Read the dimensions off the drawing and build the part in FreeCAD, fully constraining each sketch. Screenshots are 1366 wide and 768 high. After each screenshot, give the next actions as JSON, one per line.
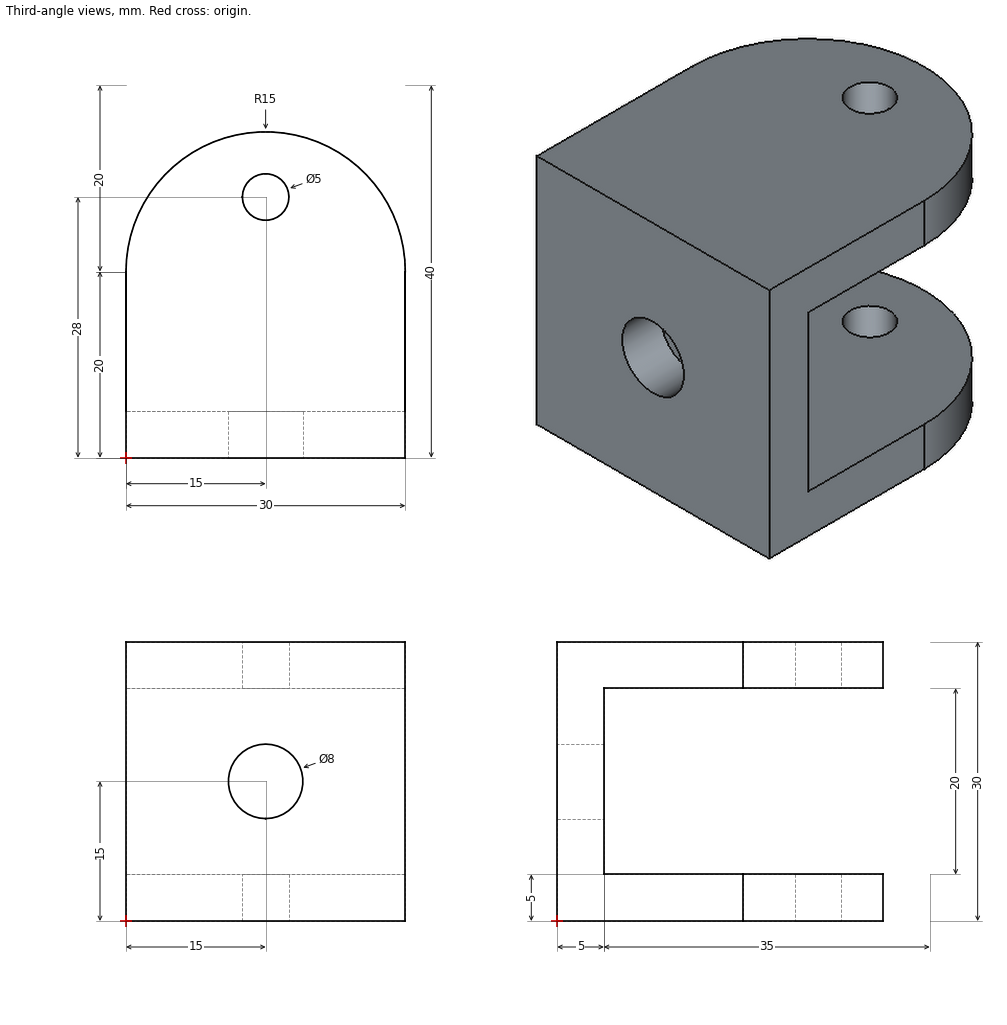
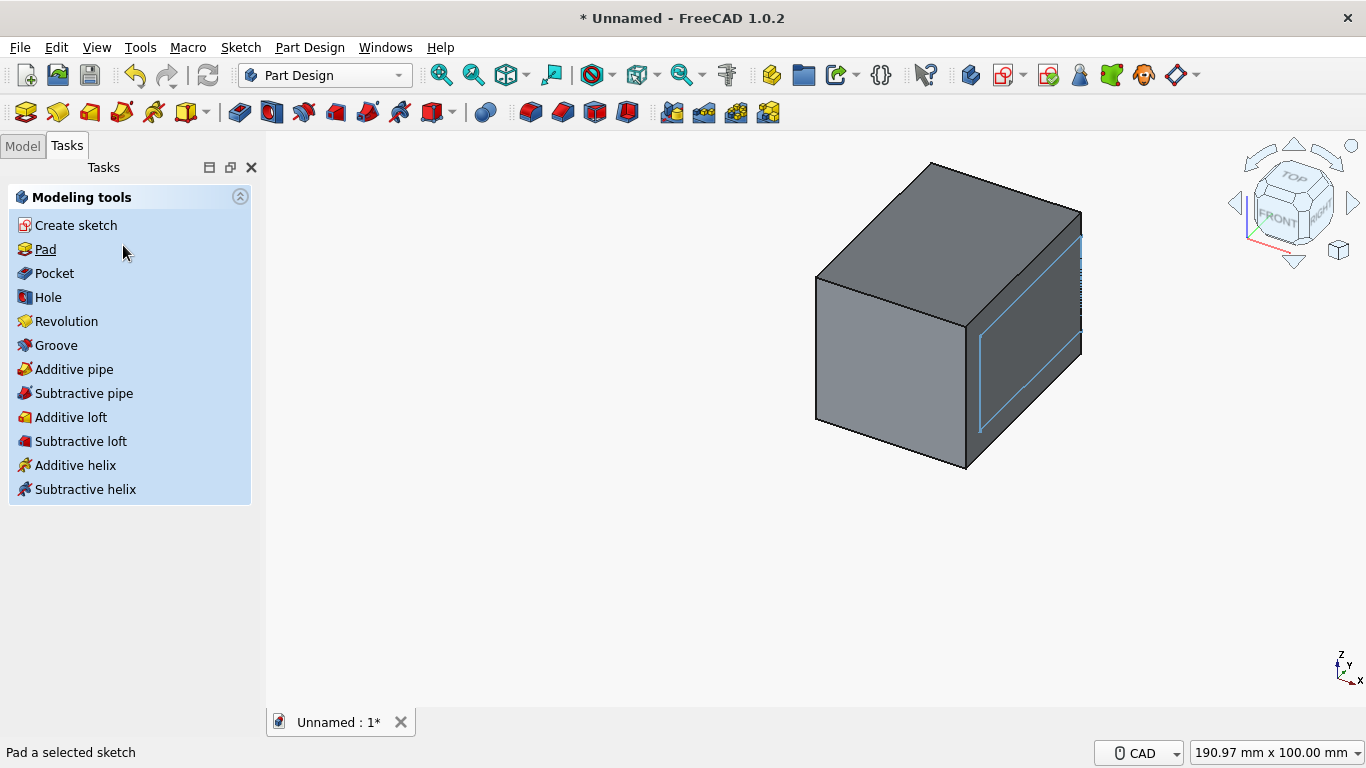
{"action": "left_click", "coordinate": [240, 112]}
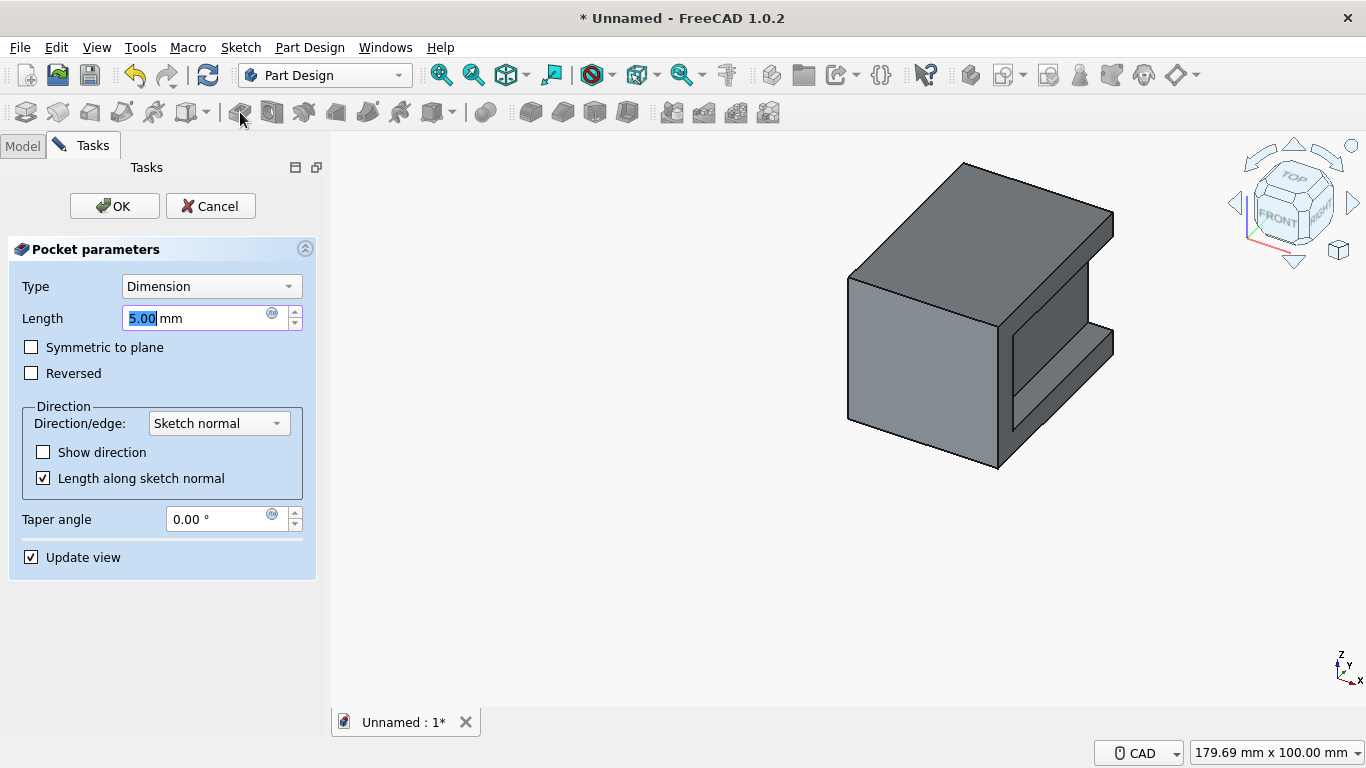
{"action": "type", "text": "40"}
{"action": "key", "text": "Tab"}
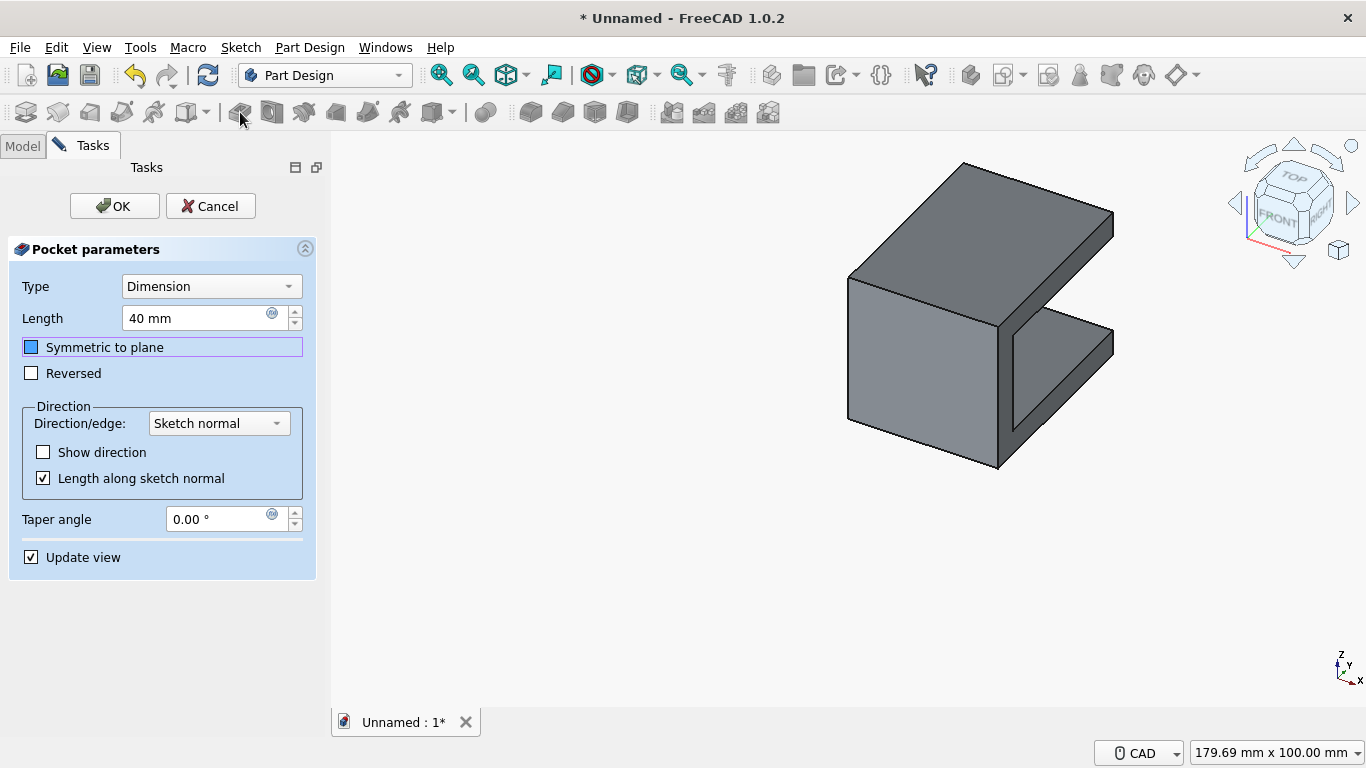
{"action": "left_click", "coordinate": [115, 206]}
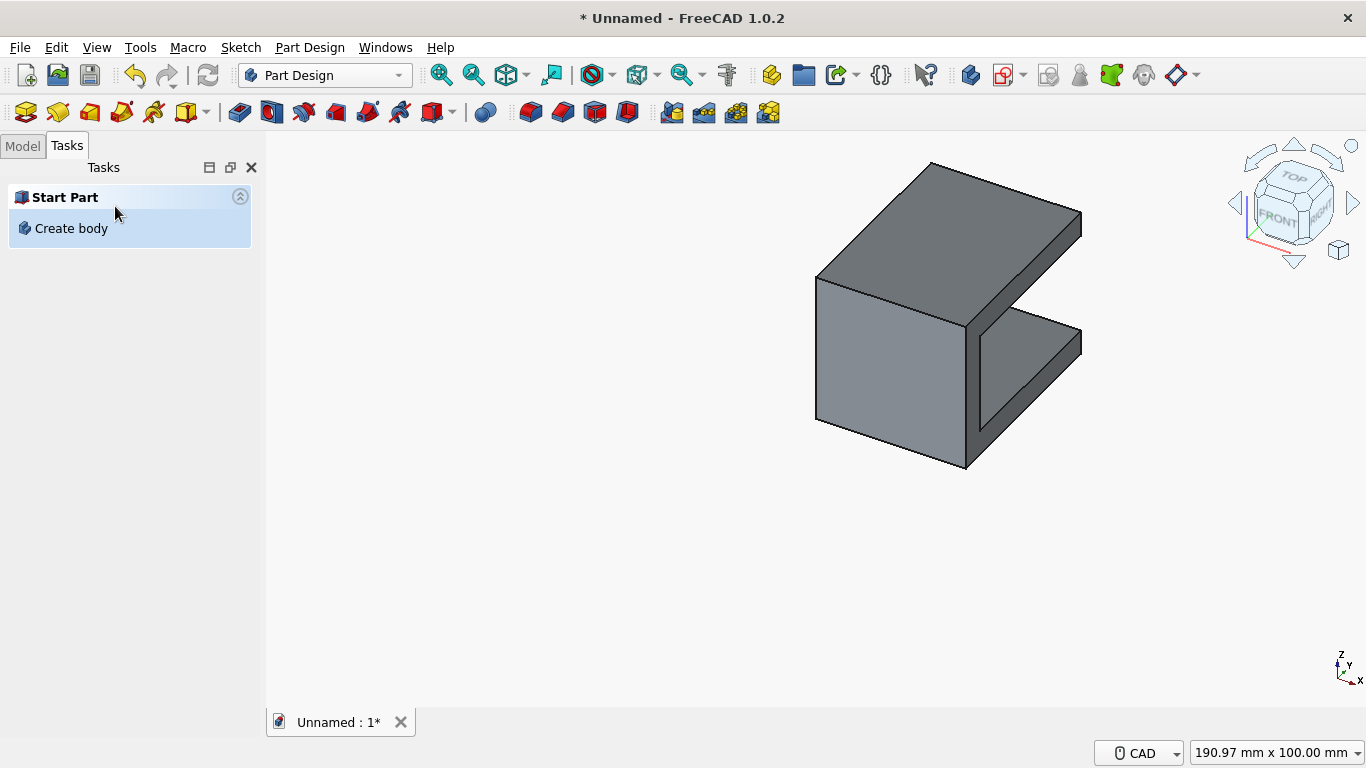
{"action": "left_click", "coordinate": [1004, 76]}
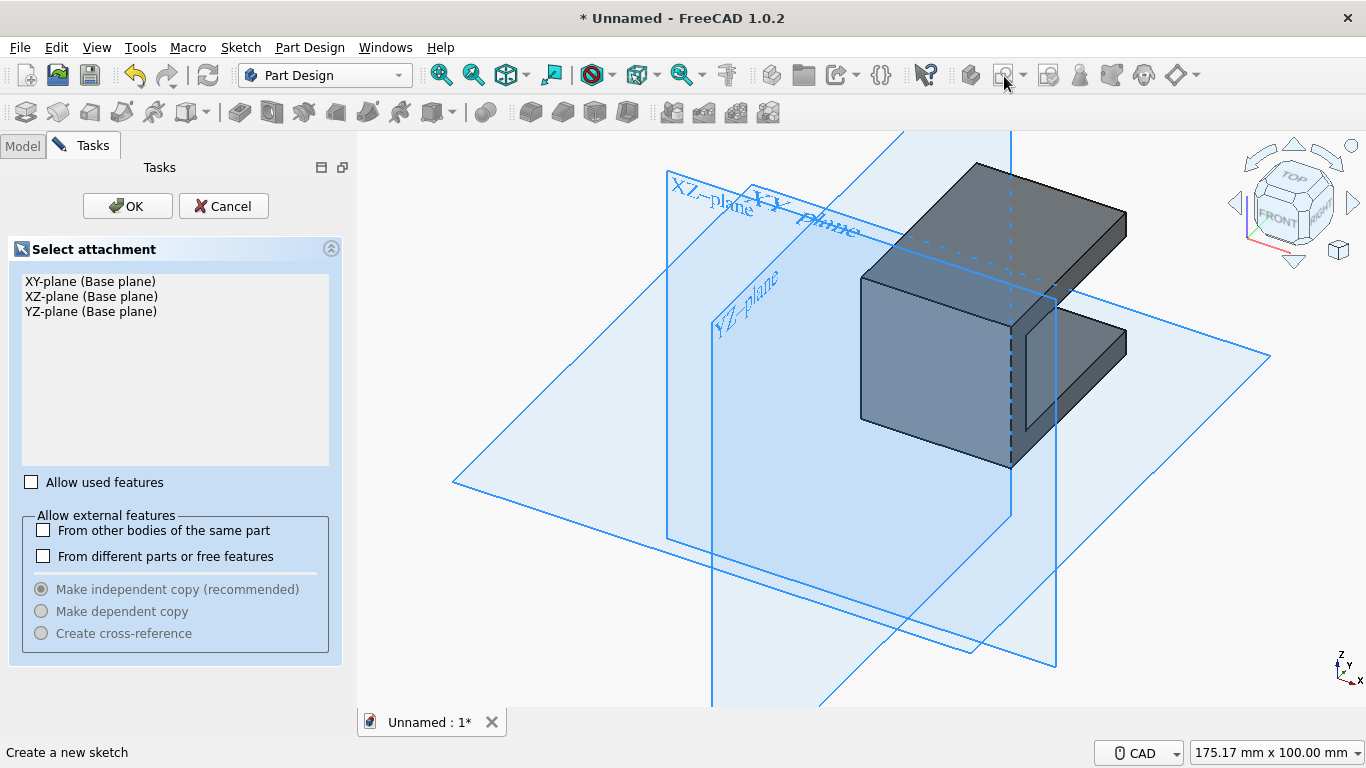
{"action": "left_click", "coordinate": [82, 282]}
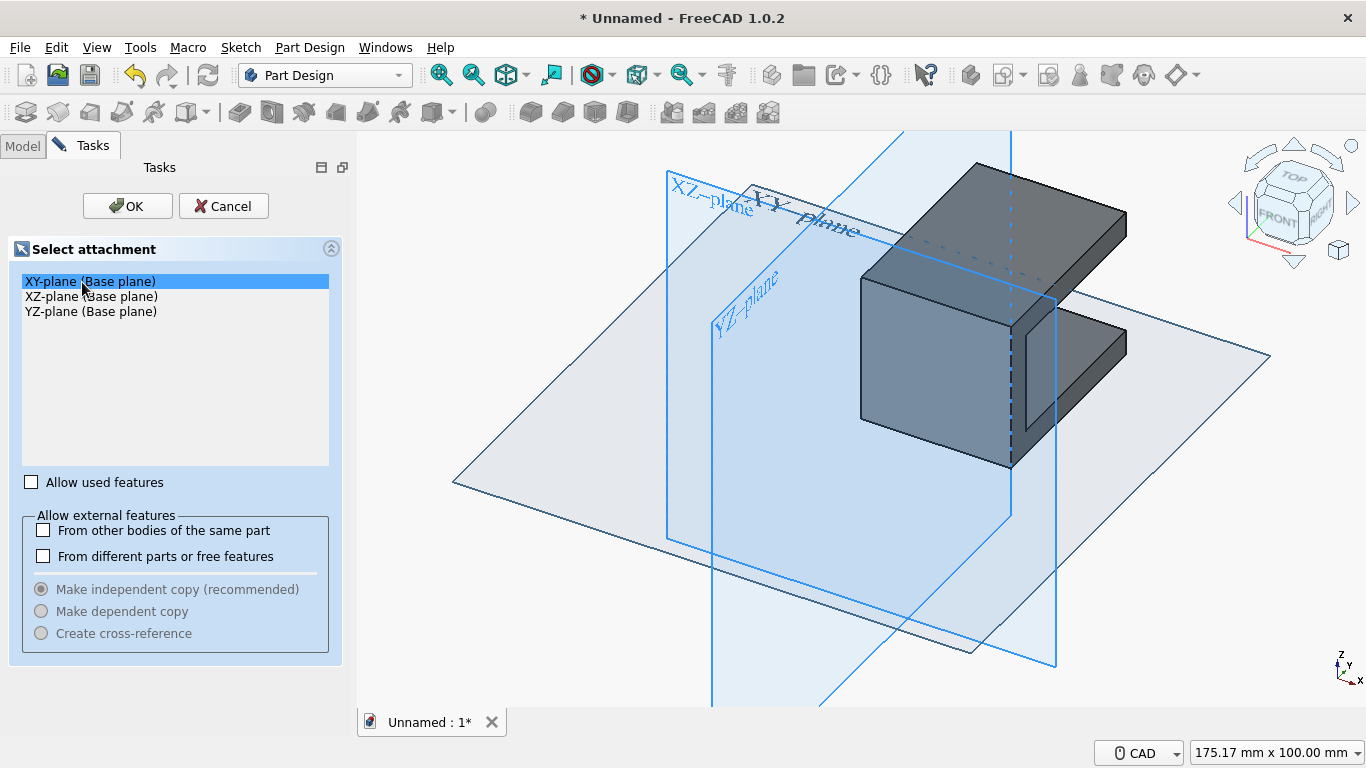
{"action": "left_click", "coordinate": [128, 206]}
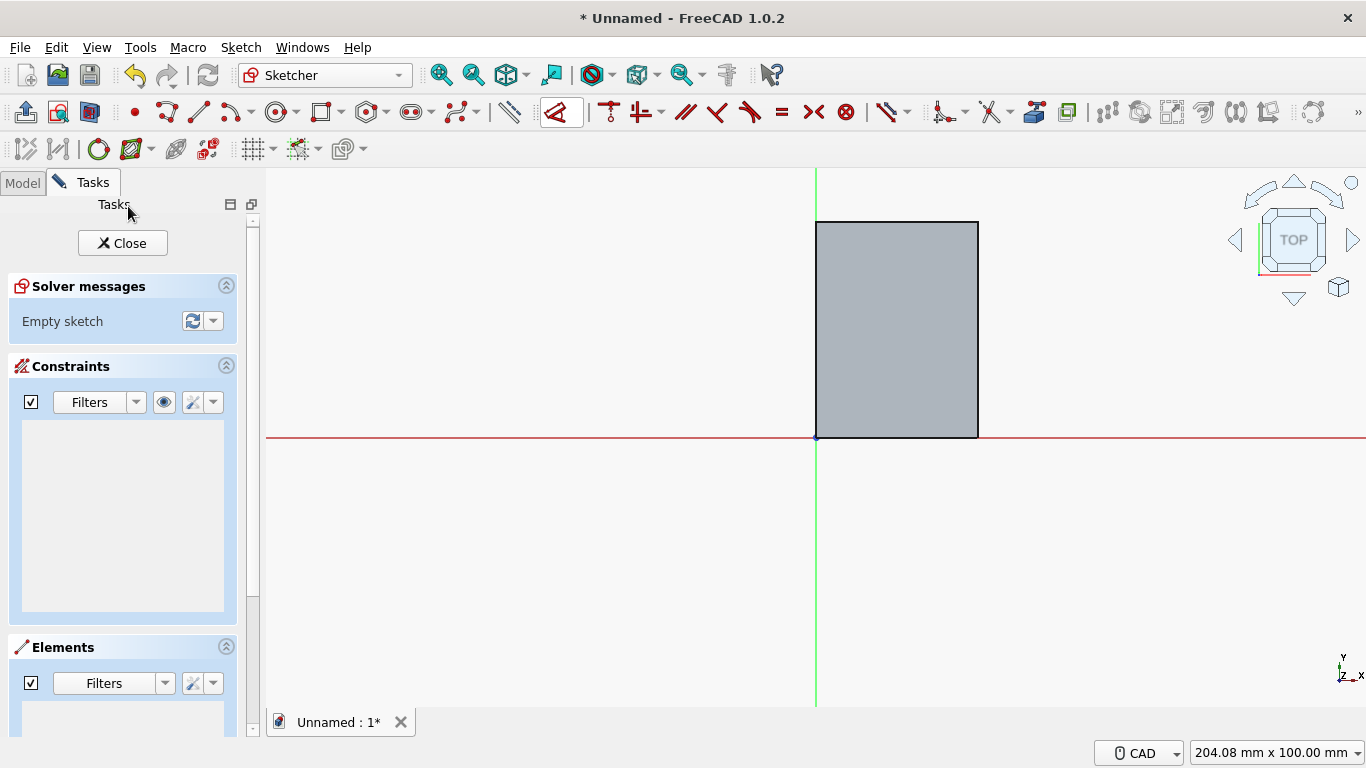
{"action": "left_click", "coordinate": [90, 112]}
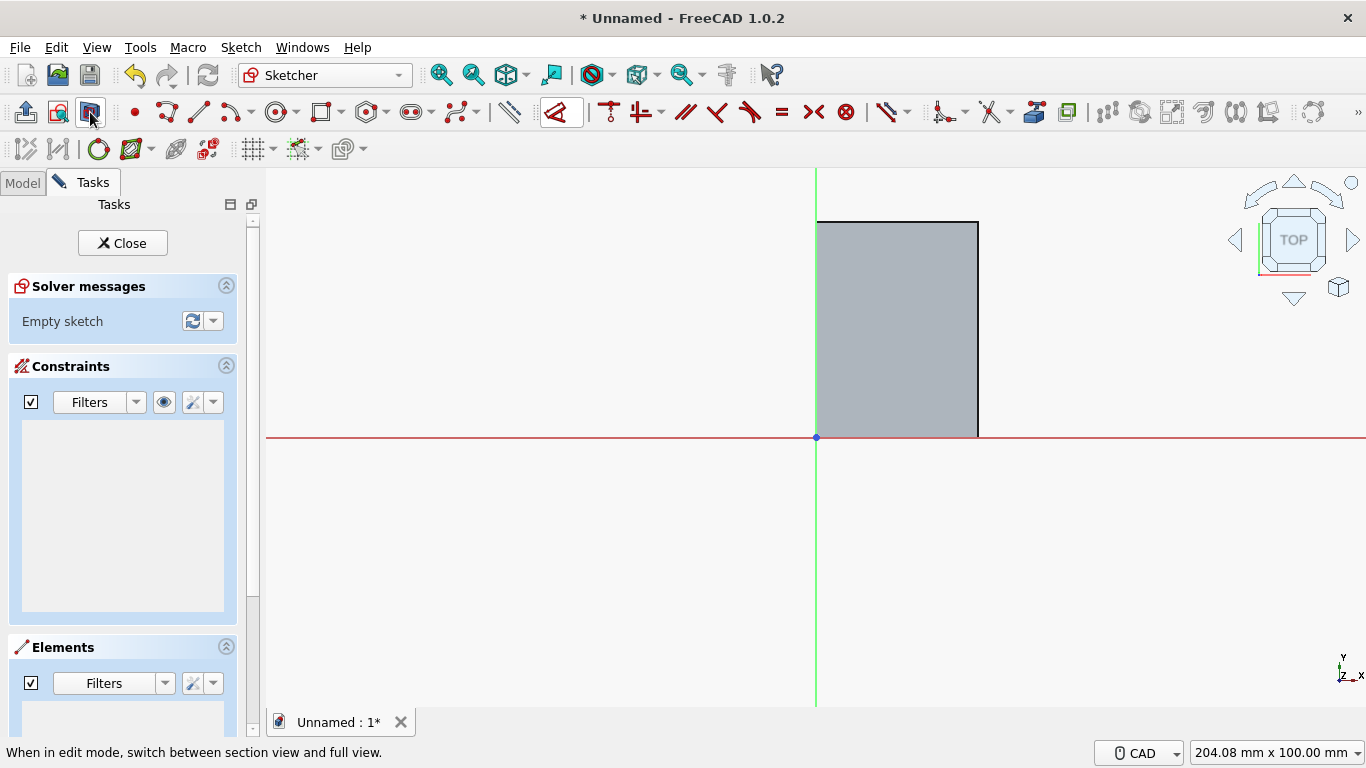
{"action": "scroll", "coordinate": [1201, 196], "scroll_direction": "up", "scroll_amount": 2}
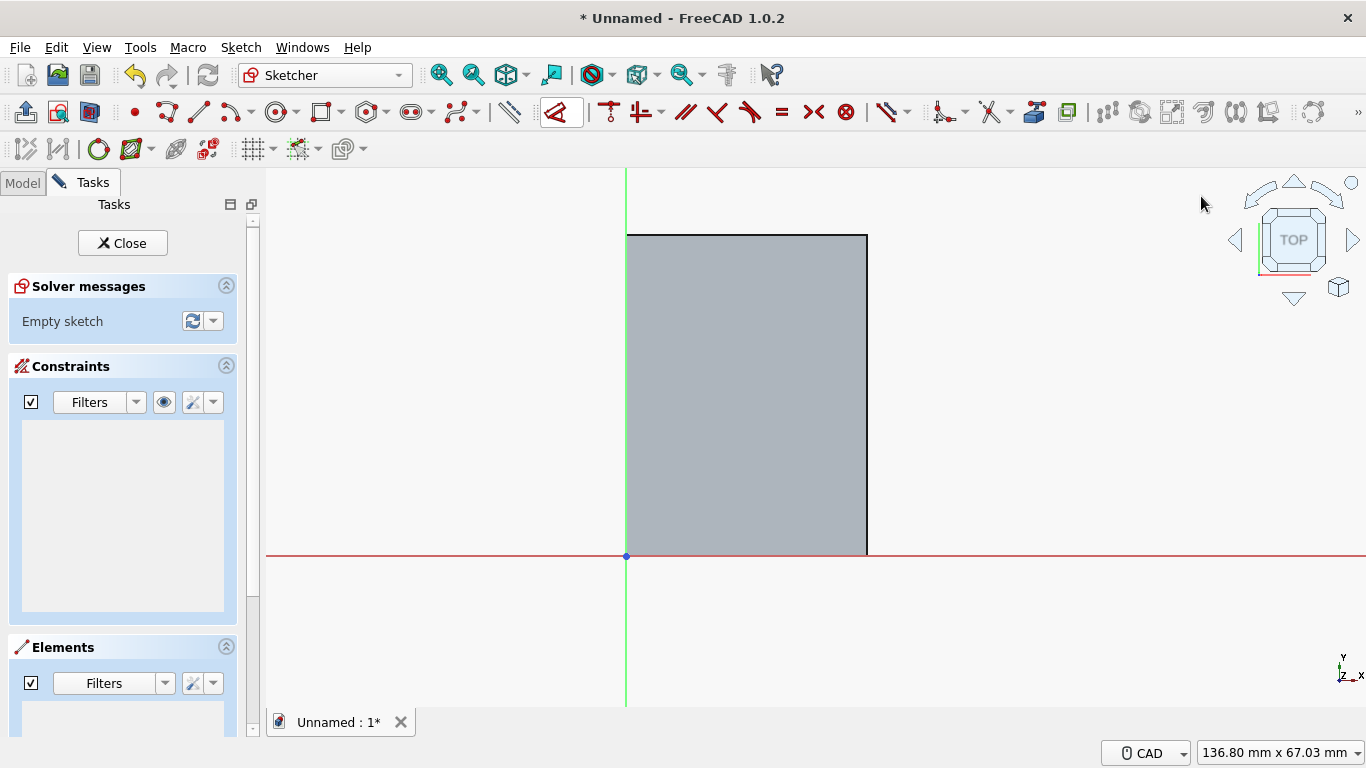
{"action": "left_click", "coordinate": [168, 112]}